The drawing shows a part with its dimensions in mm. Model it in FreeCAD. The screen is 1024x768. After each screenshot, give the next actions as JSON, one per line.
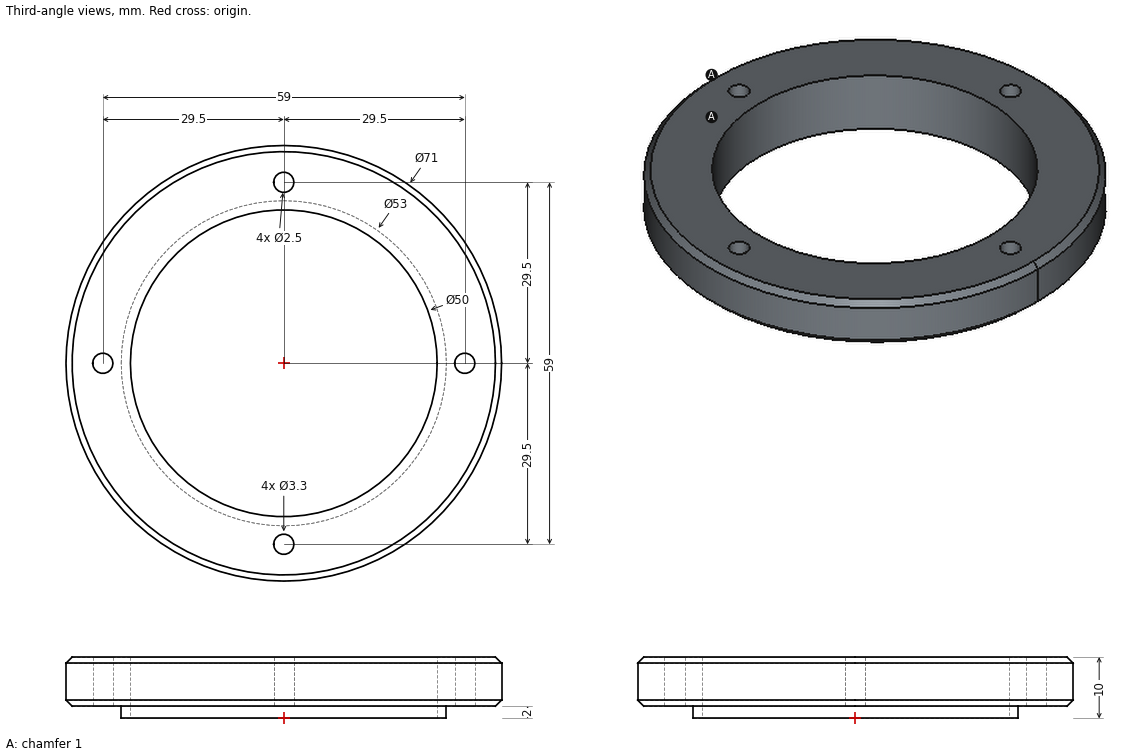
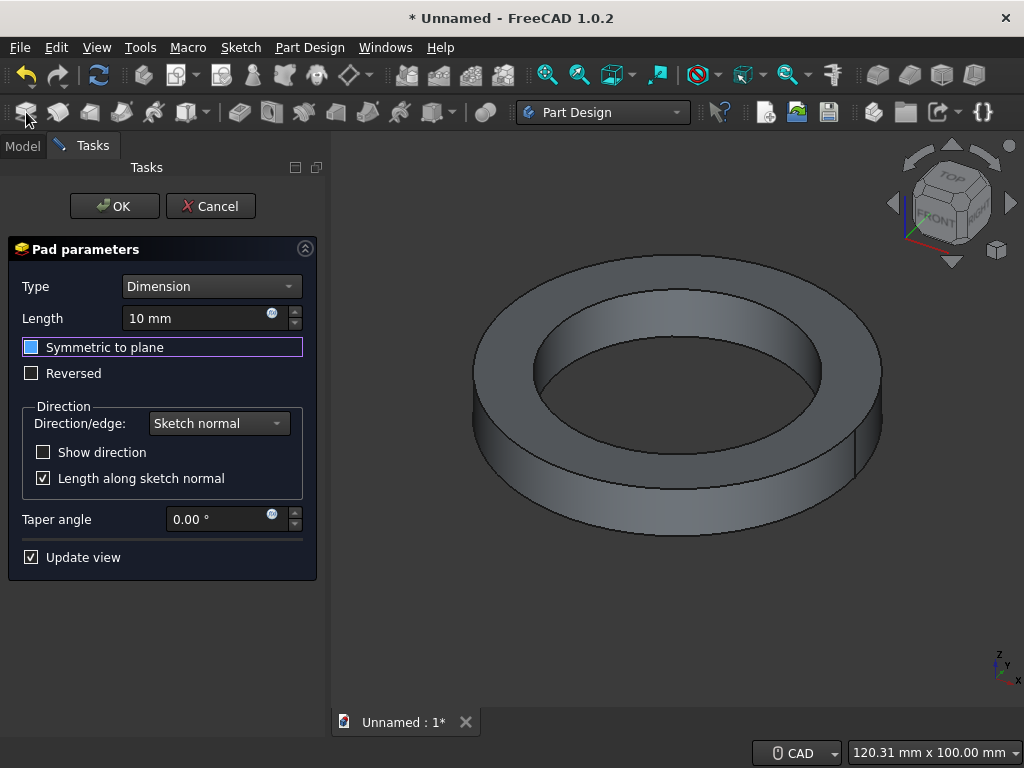
{"action": "left_click", "coordinate": [115, 206]}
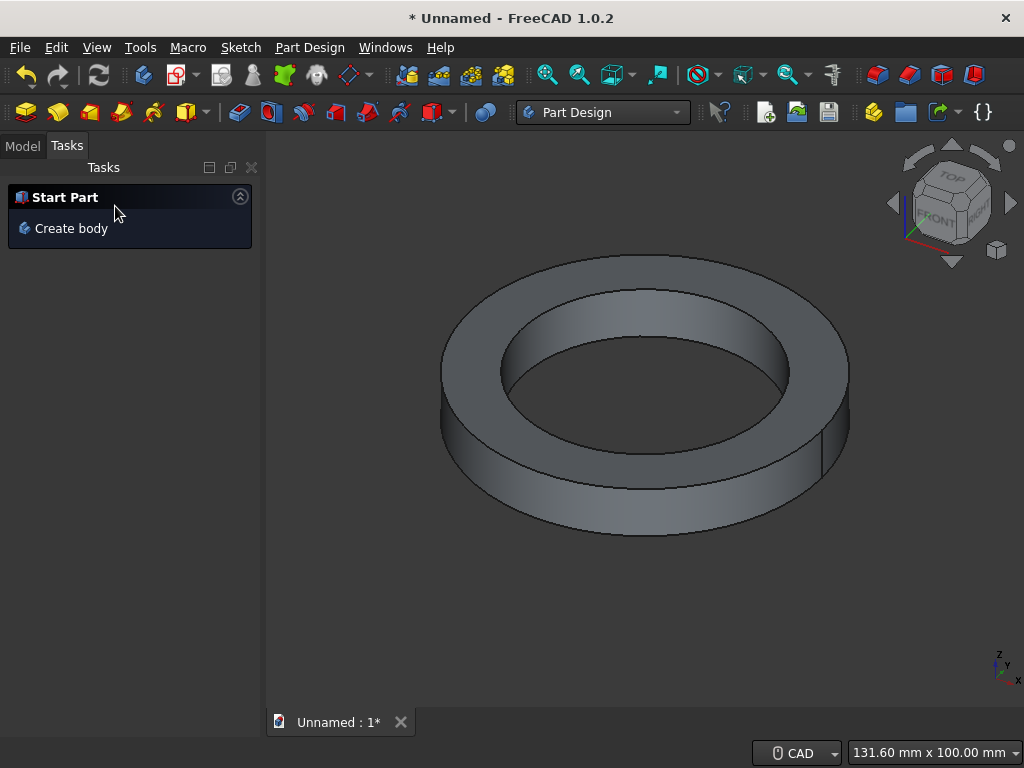
{"action": "left_click", "coordinate": [557, 458]}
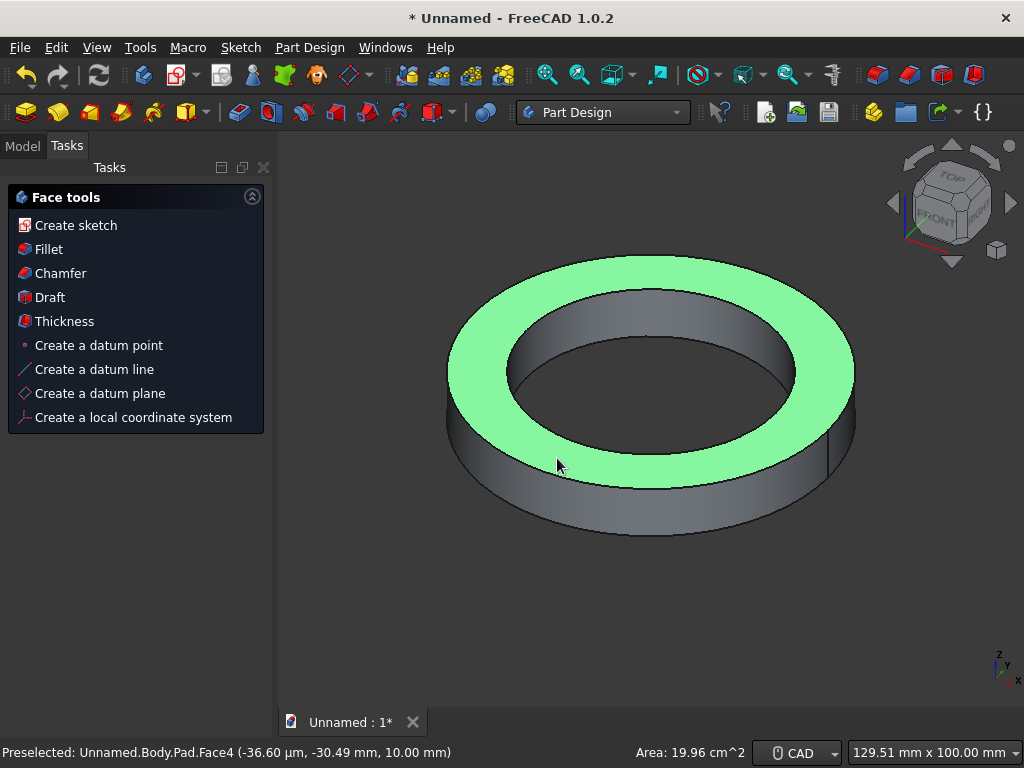
{"action": "left_click", "coordinate": [176, 76]}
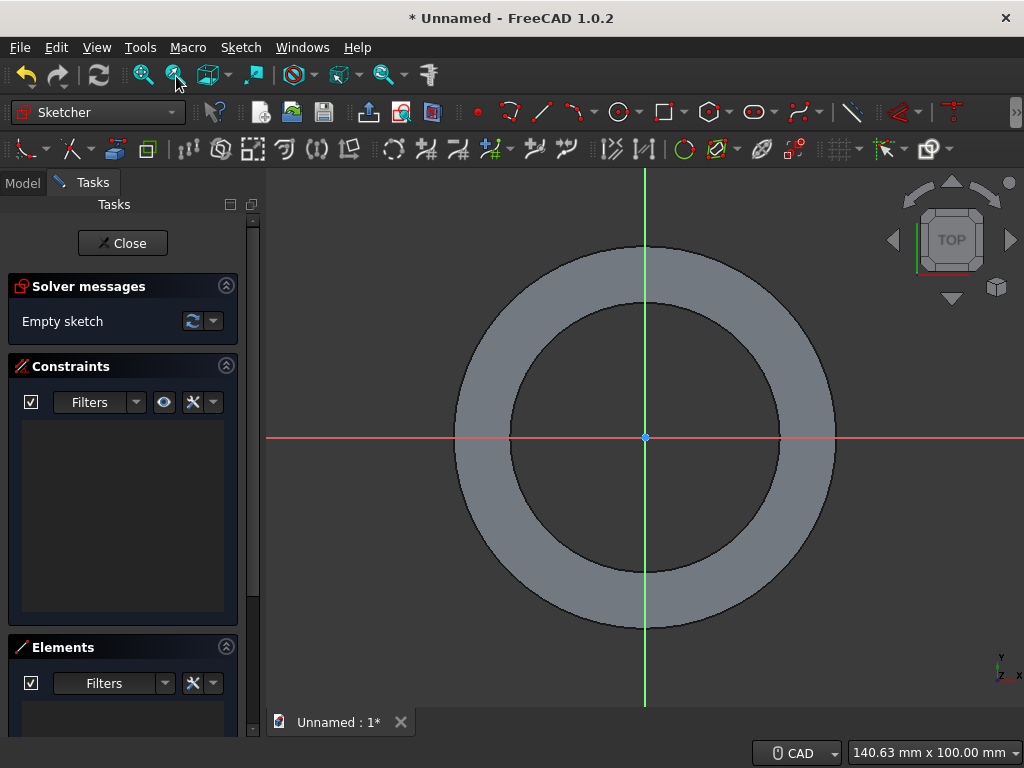
{"action": "key", "text": "g c"}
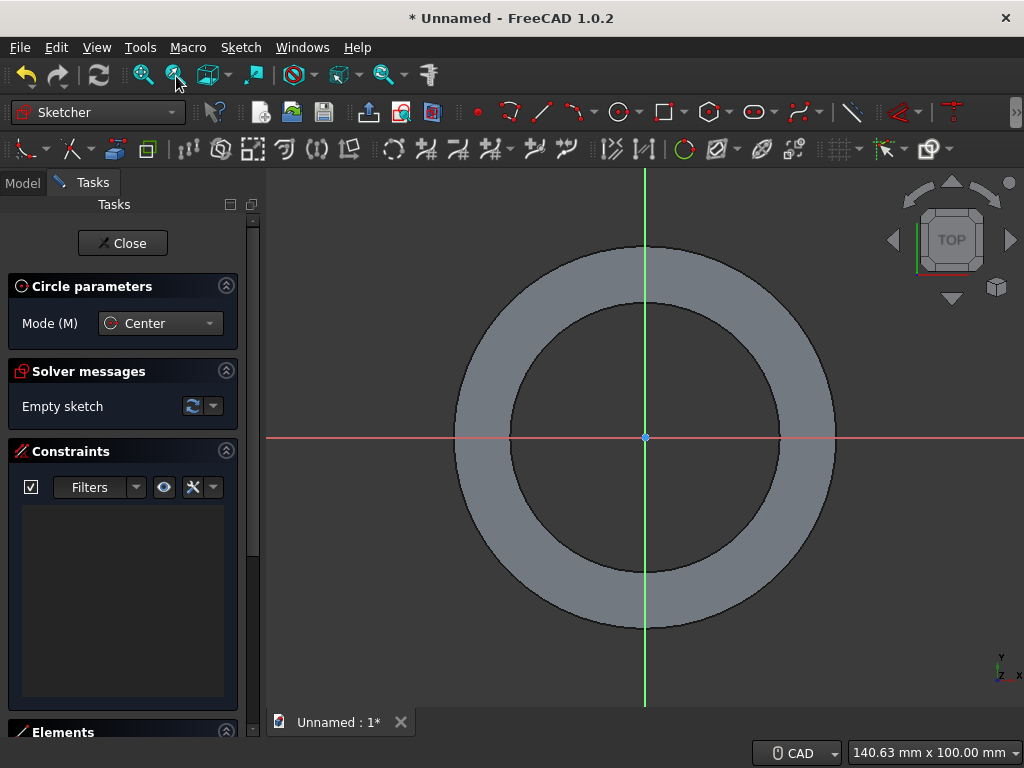
{"action": "scroll", "coordinate": [645, 278], "scroll_direction": "up", "scroll_amount": 7}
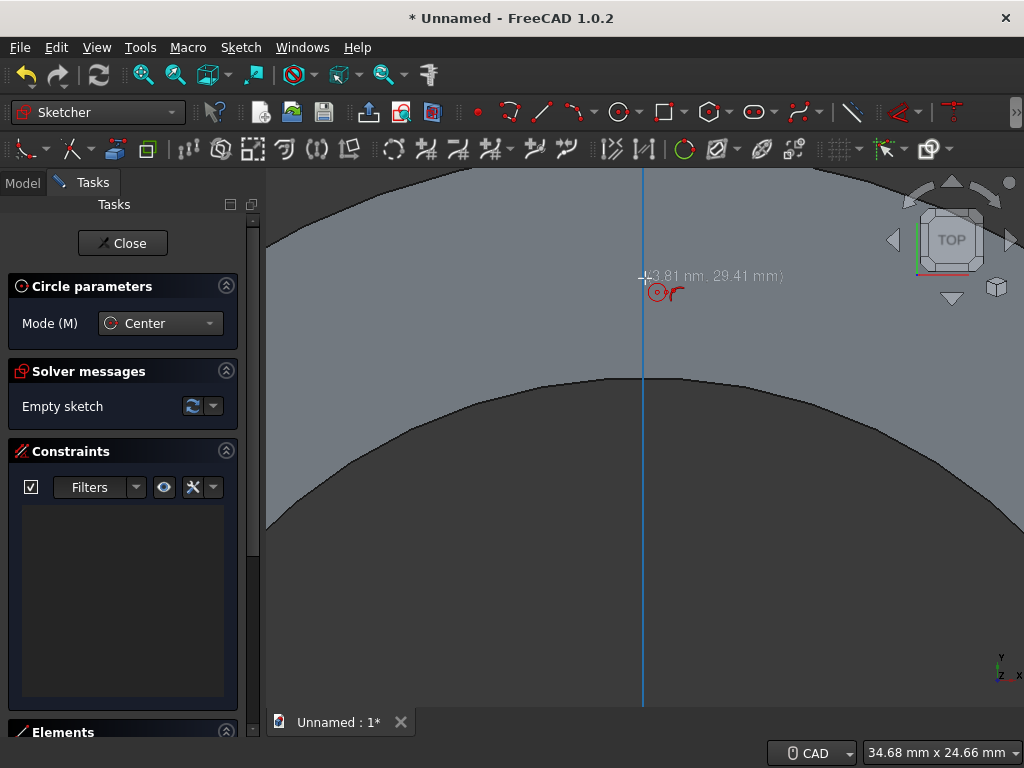
{"action": "scroll", "coordinate": [555, 278], "scroll_direction": "down", "scroll_amount": 7}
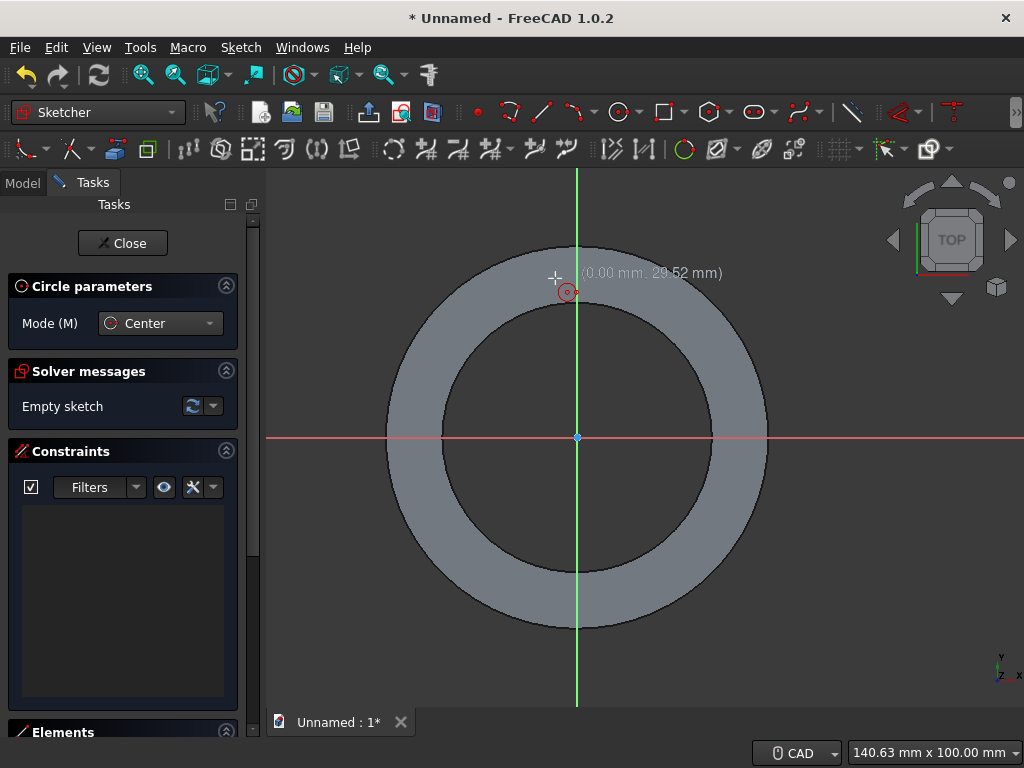
{"action": "left_click", "coordinate": [577, 278]}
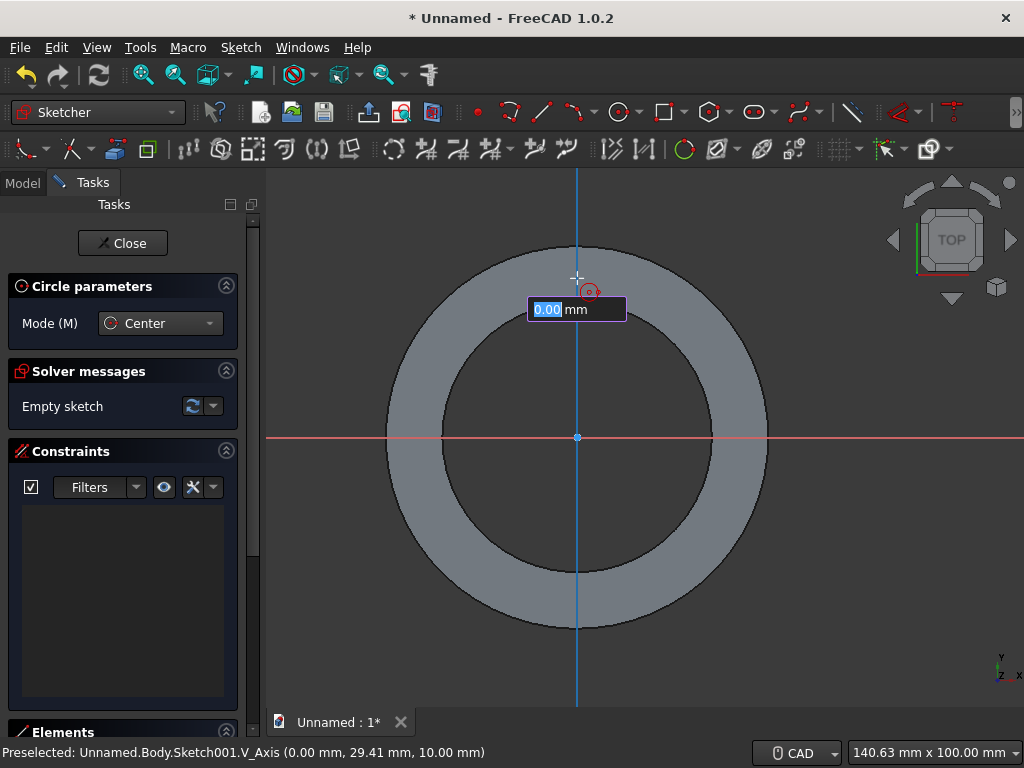
{"action": "scroll", "coordinate": [583, 276], "scroll_direction": "up", "scroll_amount": 5}
{"action": "mouse_move", "coordinate": [583, 276]}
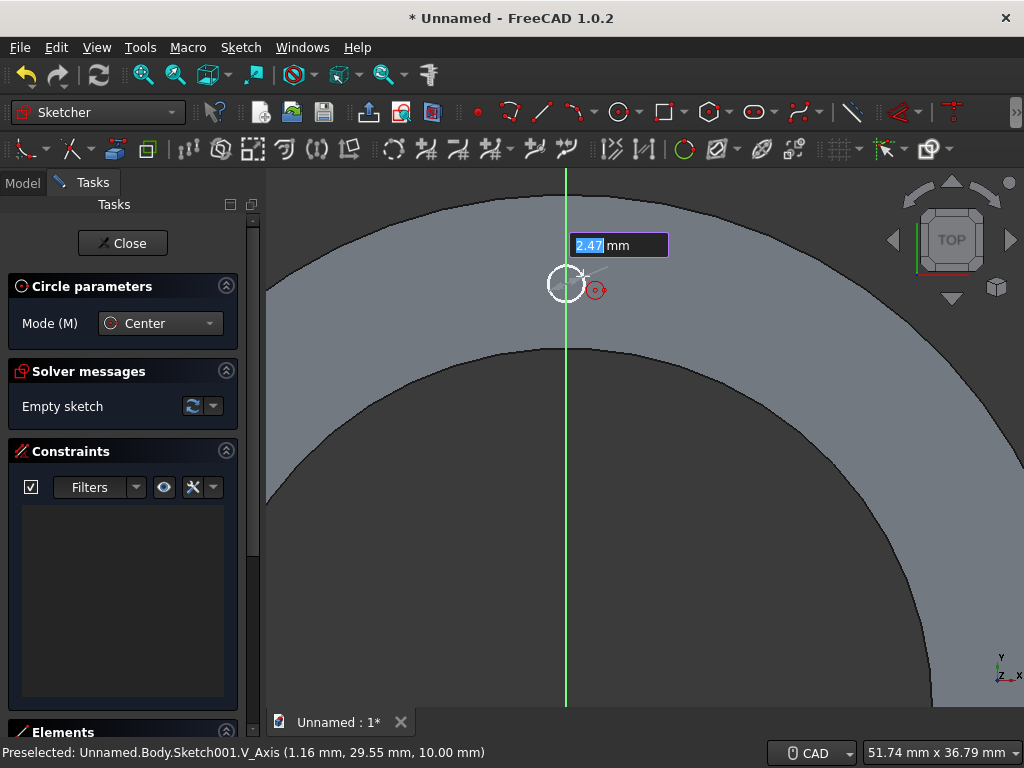
{"action": "type", "text": "2.5"}
{"action": "key", "text": "Return"}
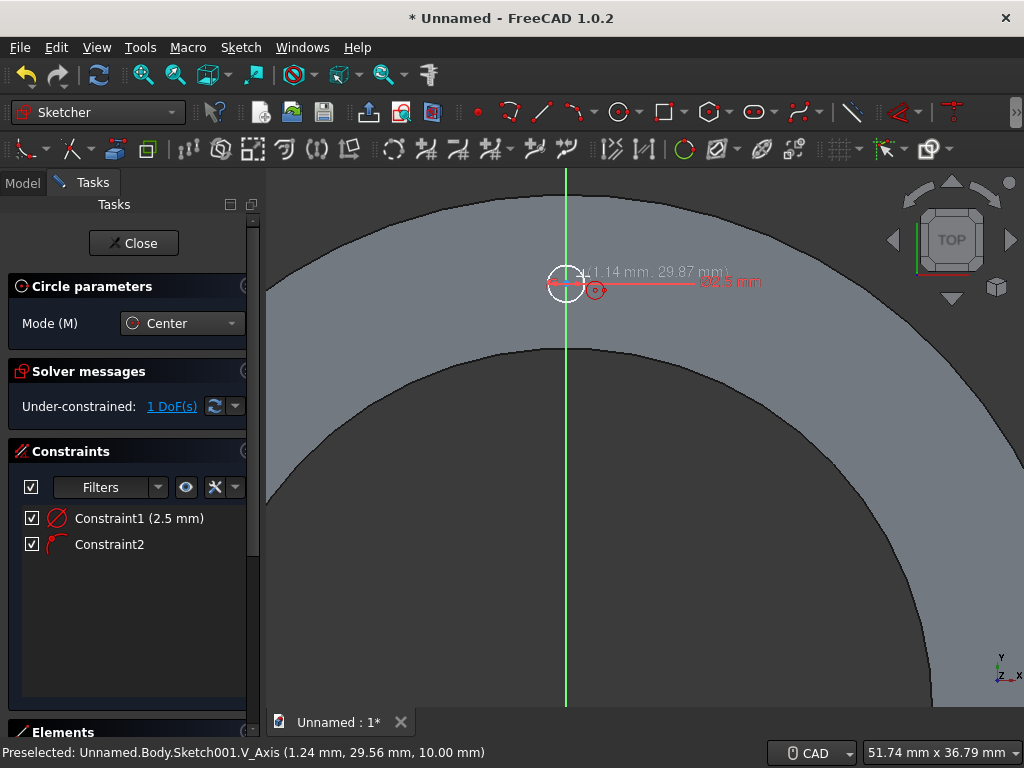
{"action": "scroll", "coordinate": [582, 276], "scroll_direction": "down", "scroll_amount": 5}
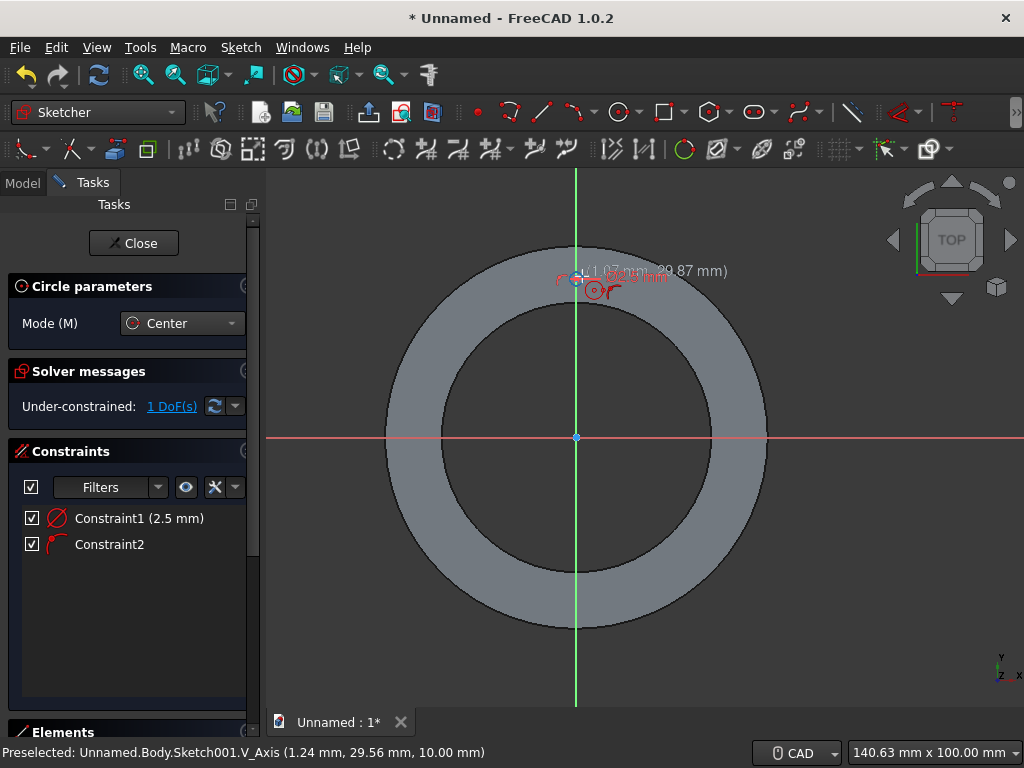
{"action": "scroll", "coordinate": [735, 437], "scroll_direction": "up", "scroll_amount": 7}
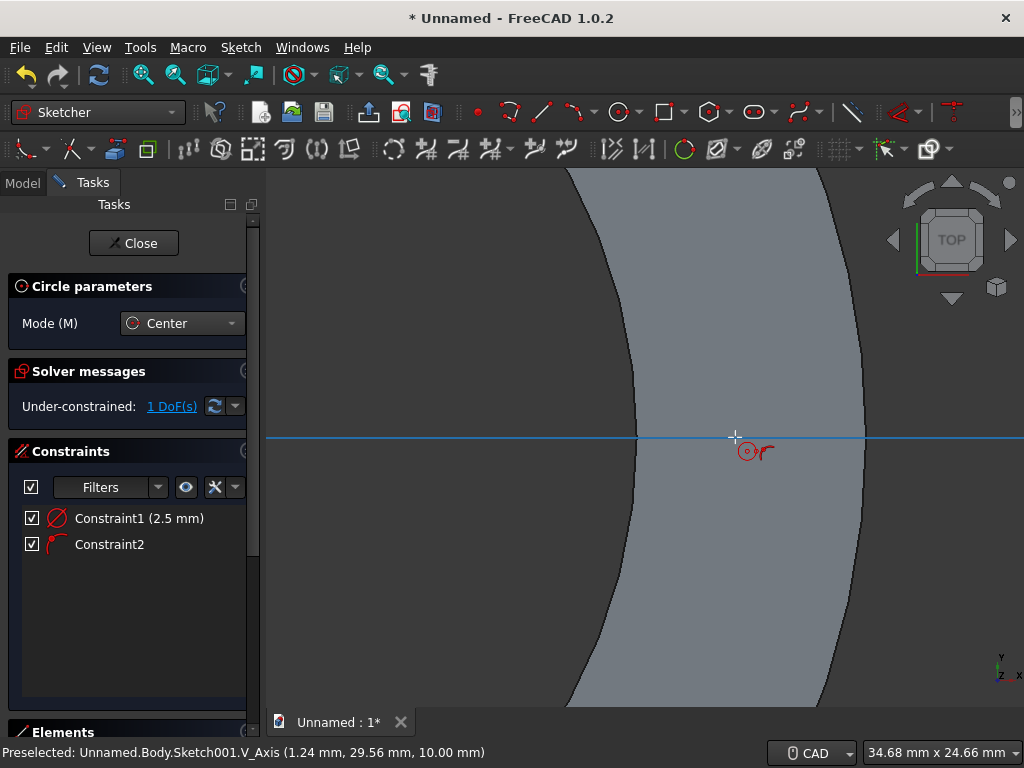
{"action": "scroll", "coordinate": [736, 438], "scroll_direction": "down", "scroll_amount": 7}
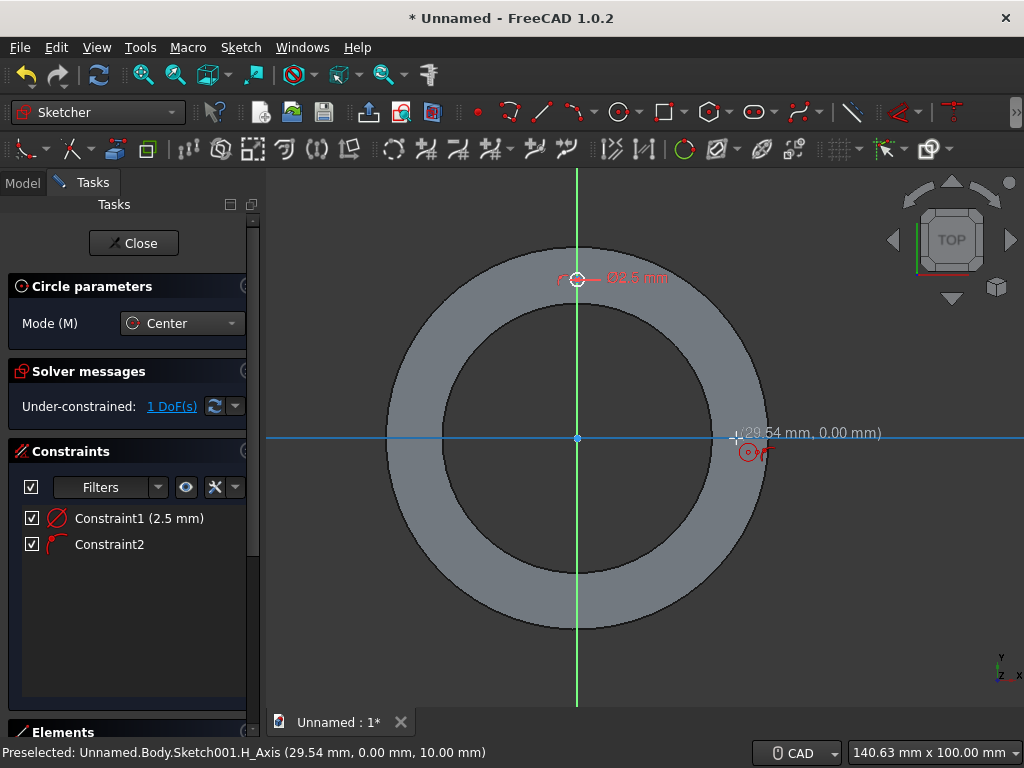
{"action": "left_click", "coordinate": [736, 438]}